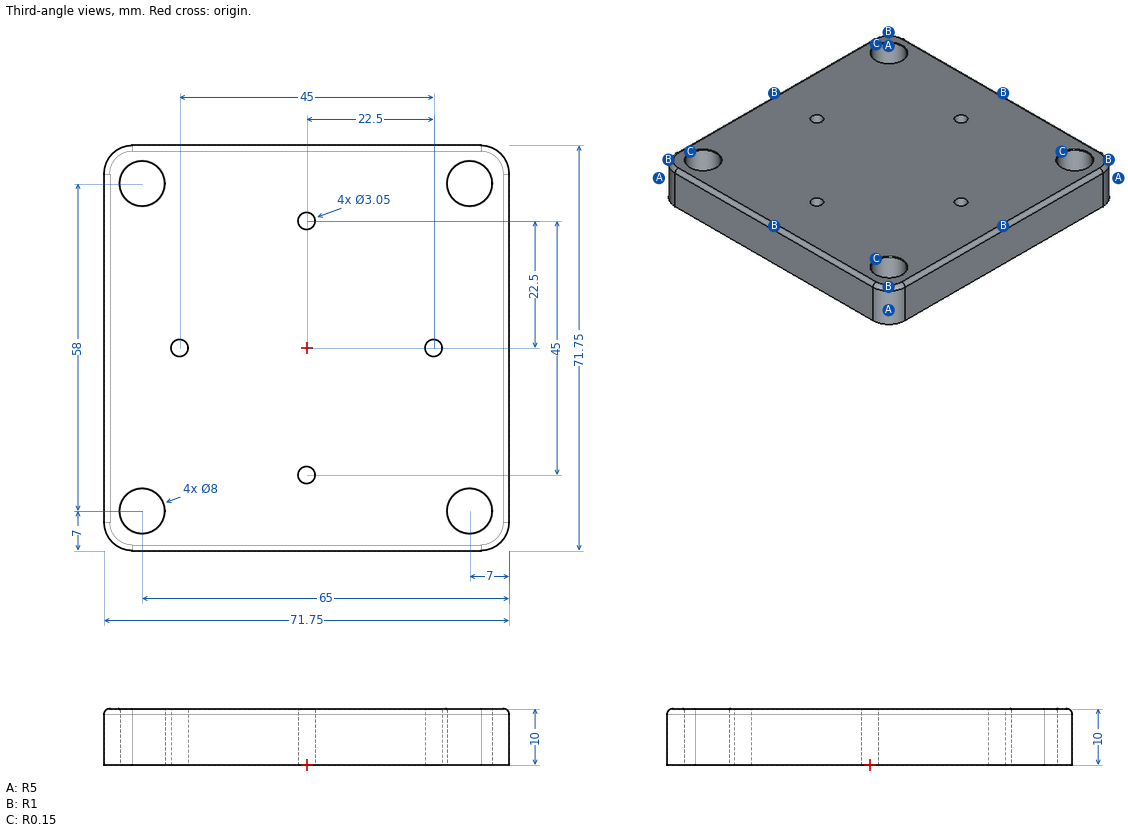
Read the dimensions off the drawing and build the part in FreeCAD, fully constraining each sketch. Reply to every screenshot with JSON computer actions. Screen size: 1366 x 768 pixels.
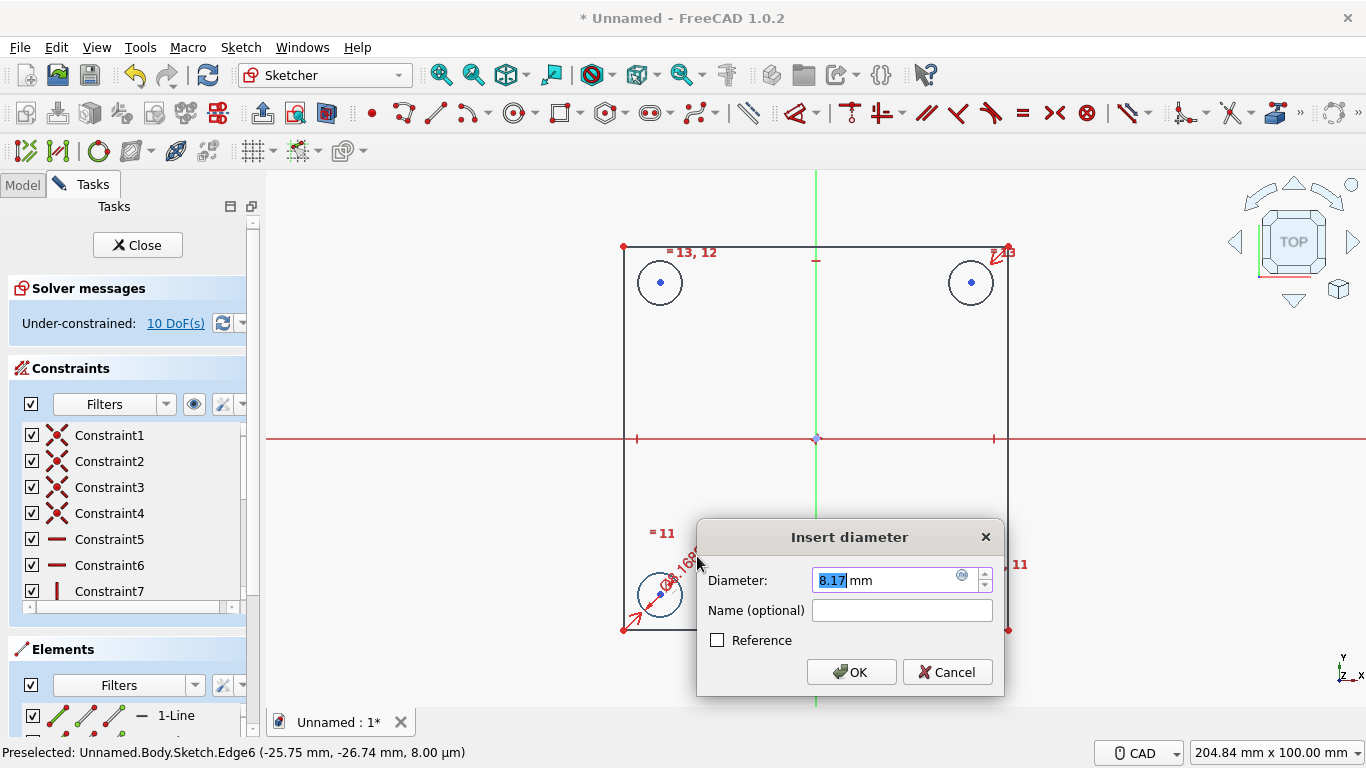
{"action": "type", "text": "8"}
{"action": "key", "text": "Return"}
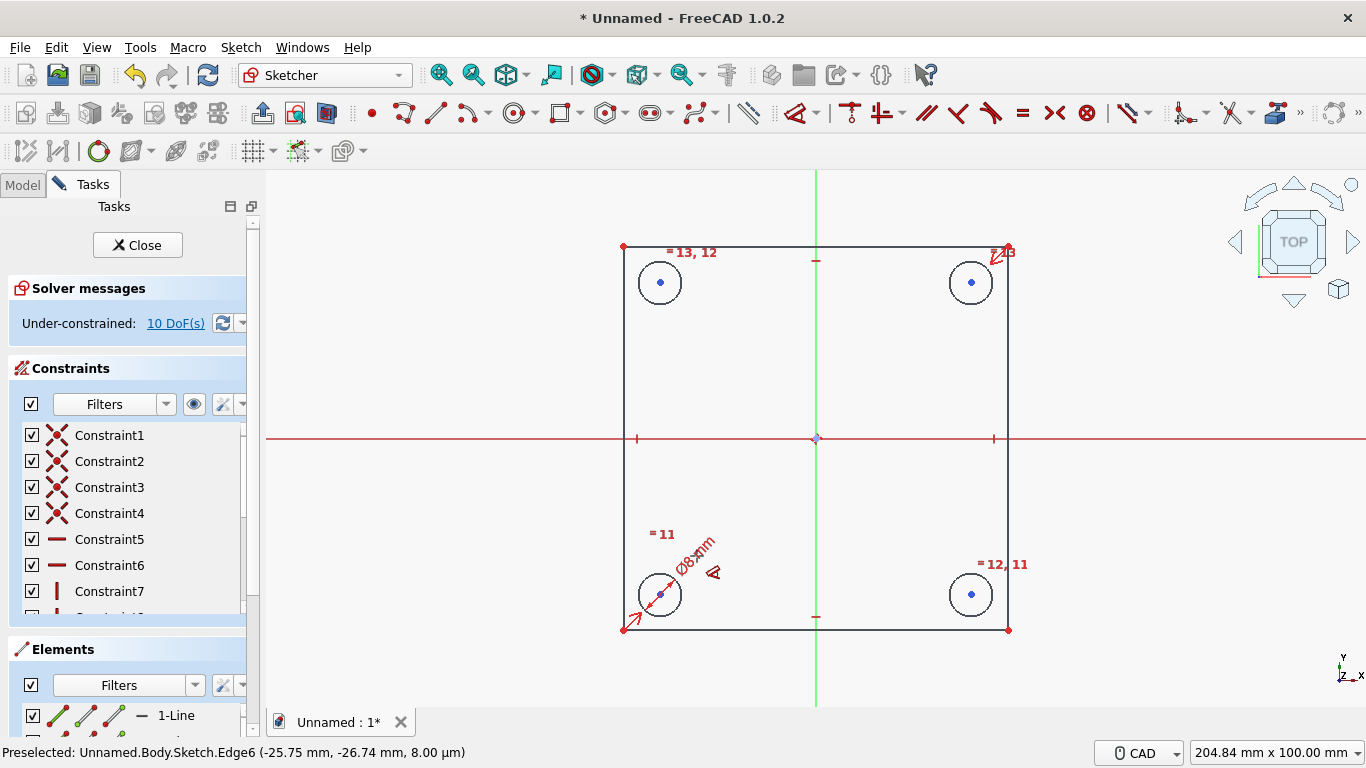
{"action": "left_click", "coordinate": [624, 630]}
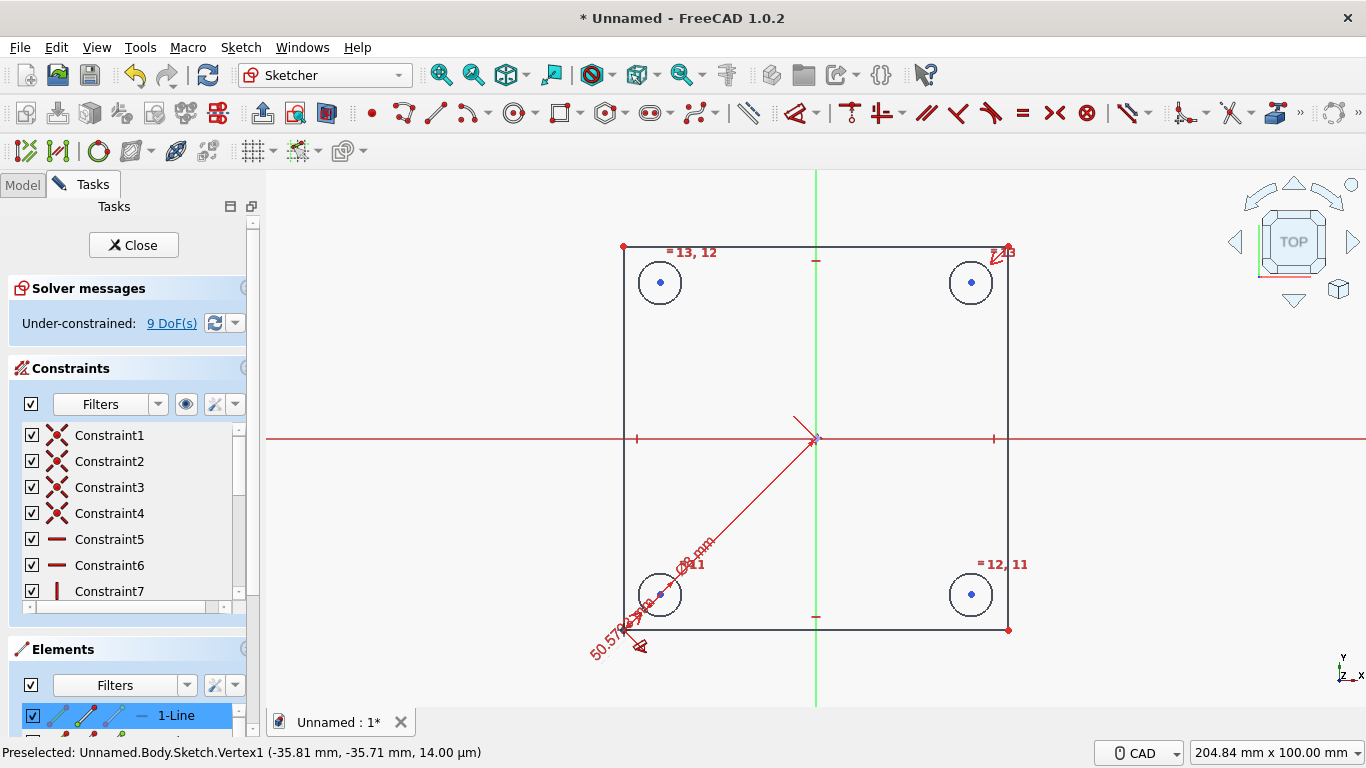
{"action": "left_click", "coordinate": [660, 595]}
{"action": "left_click", "coordinate": [590, 613]}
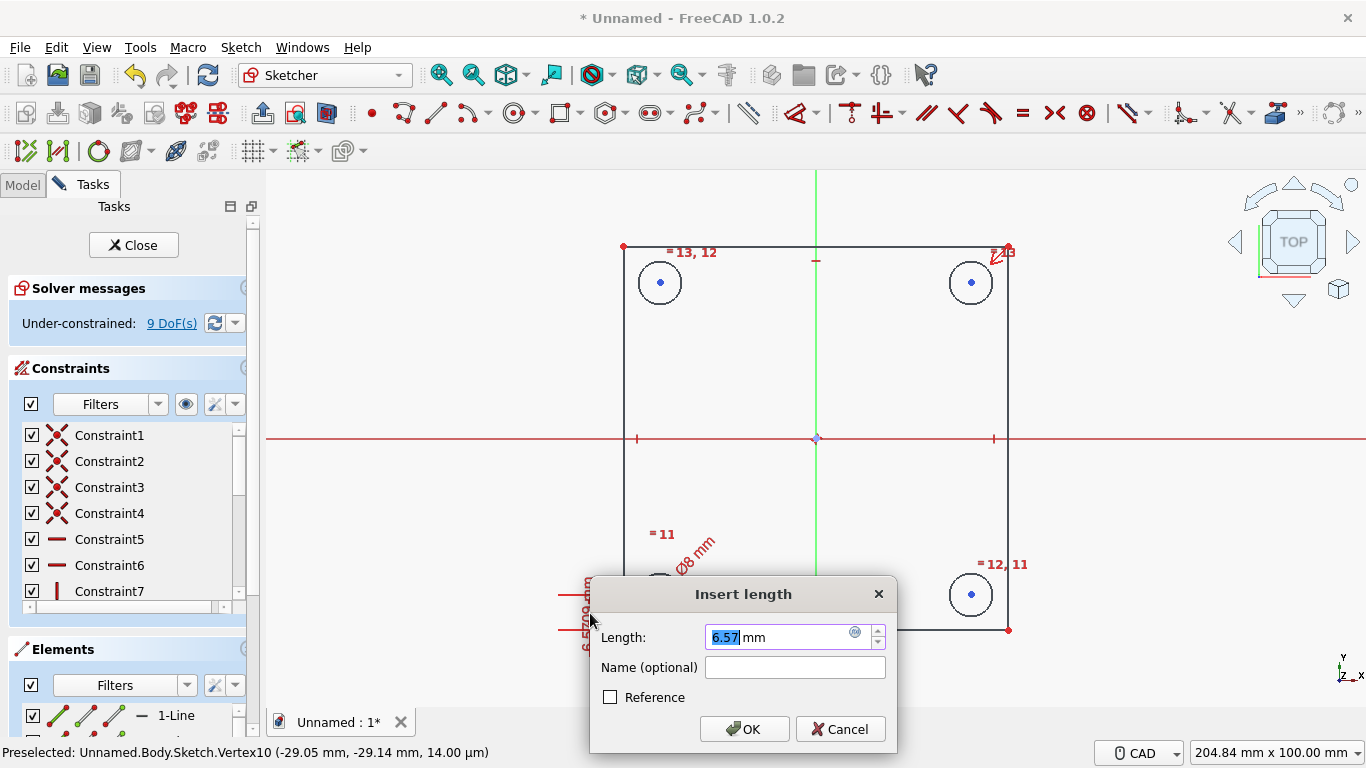
{"action": "type", "text": "7"}
{"action": "key", "text": "Return"}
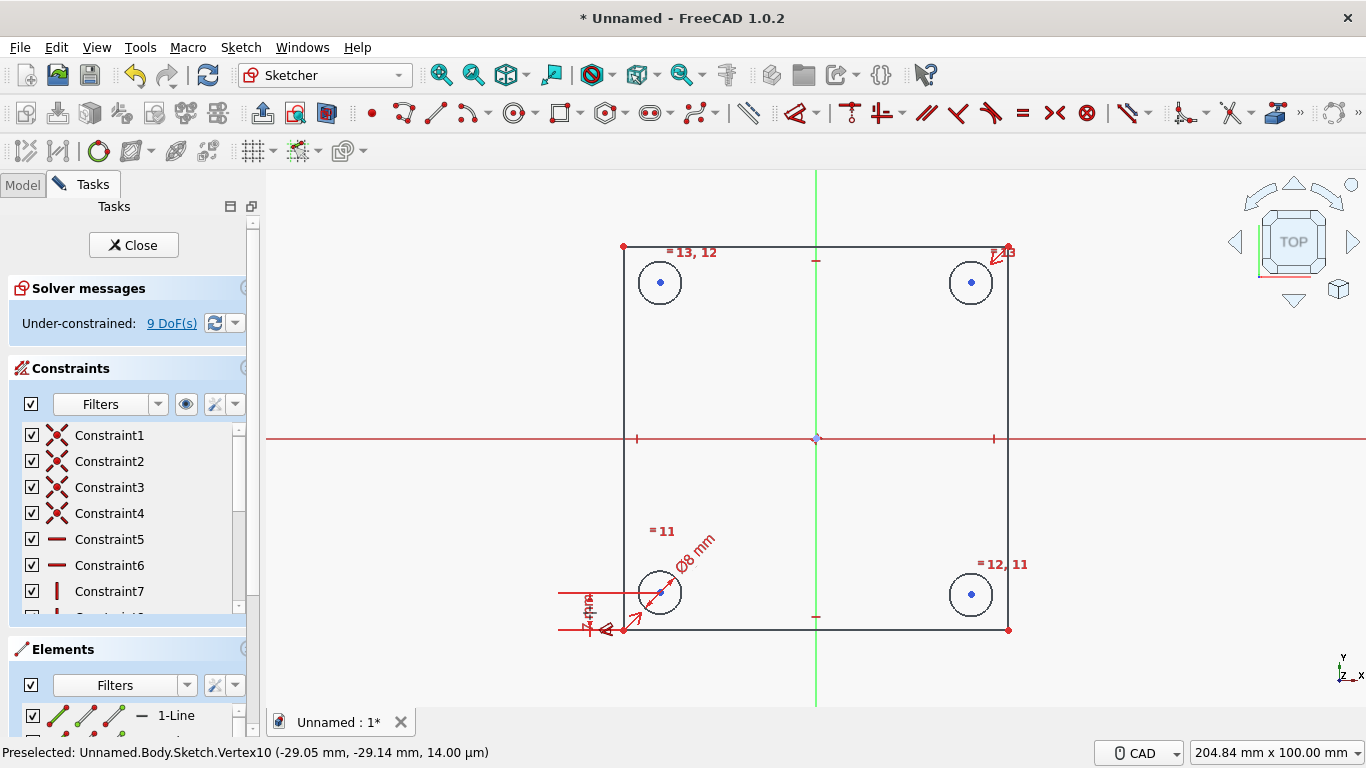
{"action": "left_click", "coordinate": [1008, 630]}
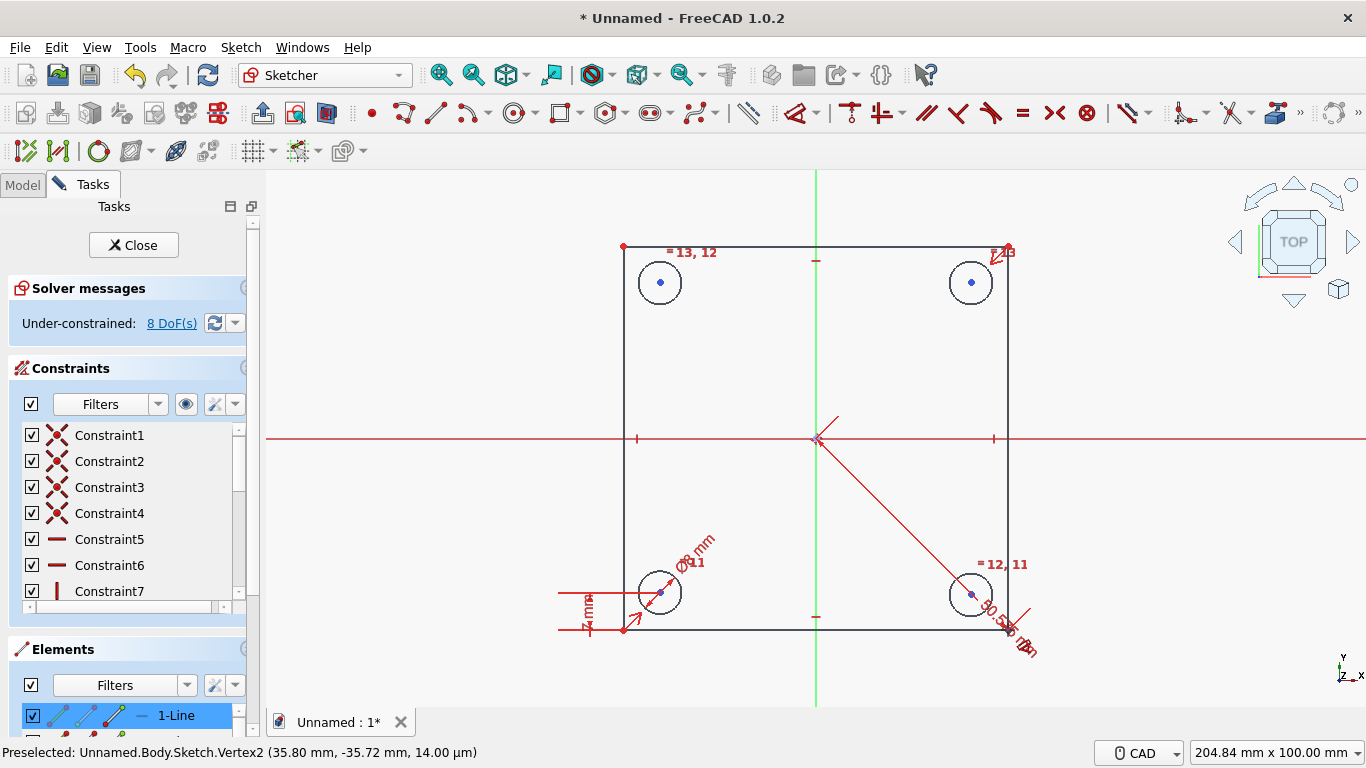
{"action": "left_click", "coordinate": [971, 595]}
{"action": "left_click", "coordinate": [990, 664]}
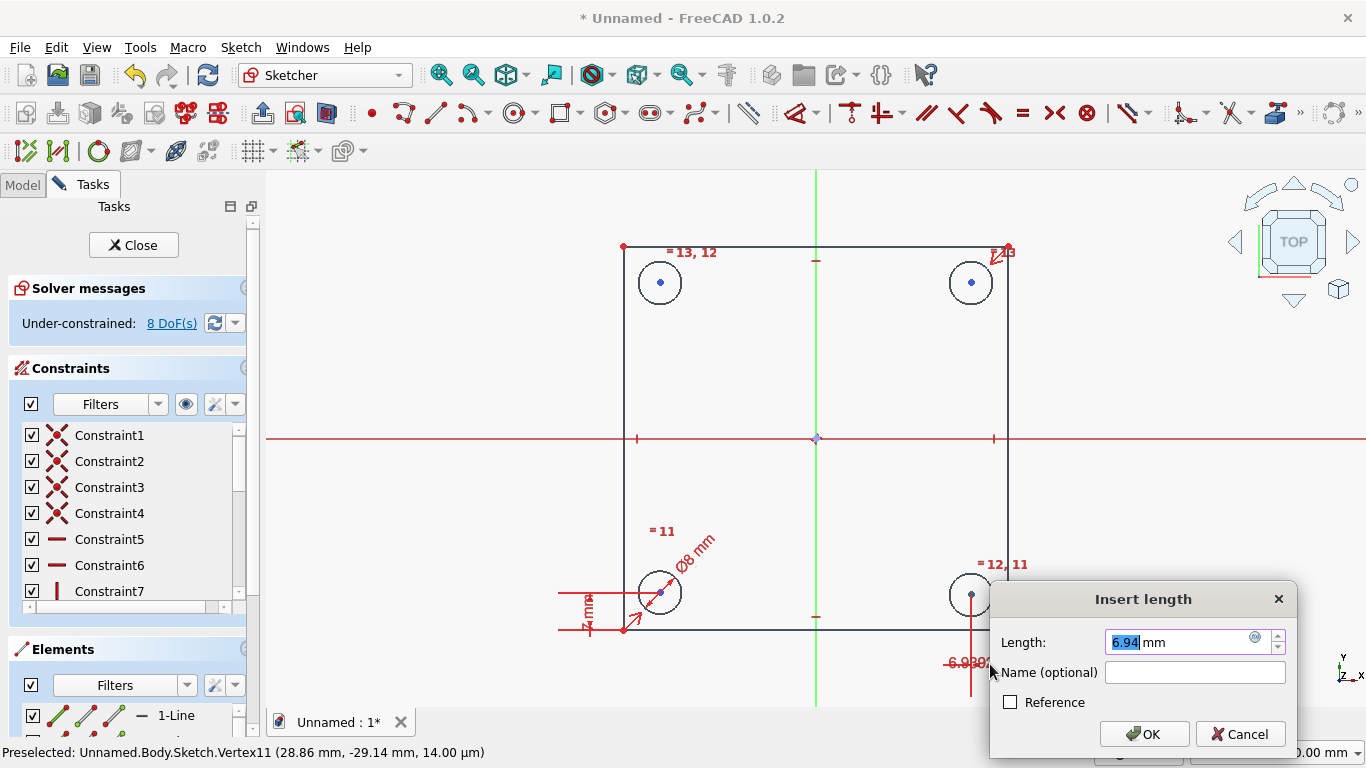
{"action": "type", "text": "7"}
{"action": "key", "text": "Return"}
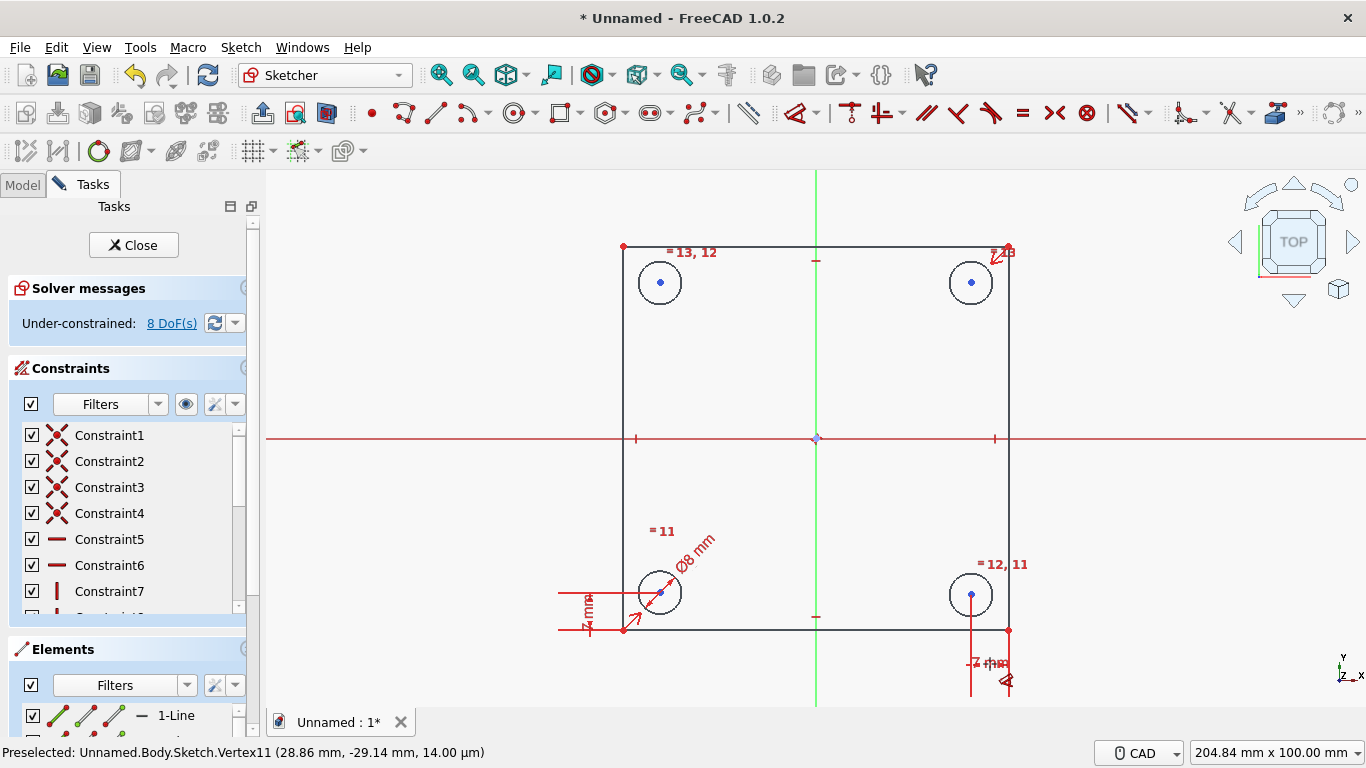
{"action": "left_click", "coordinate": [1009, 630]}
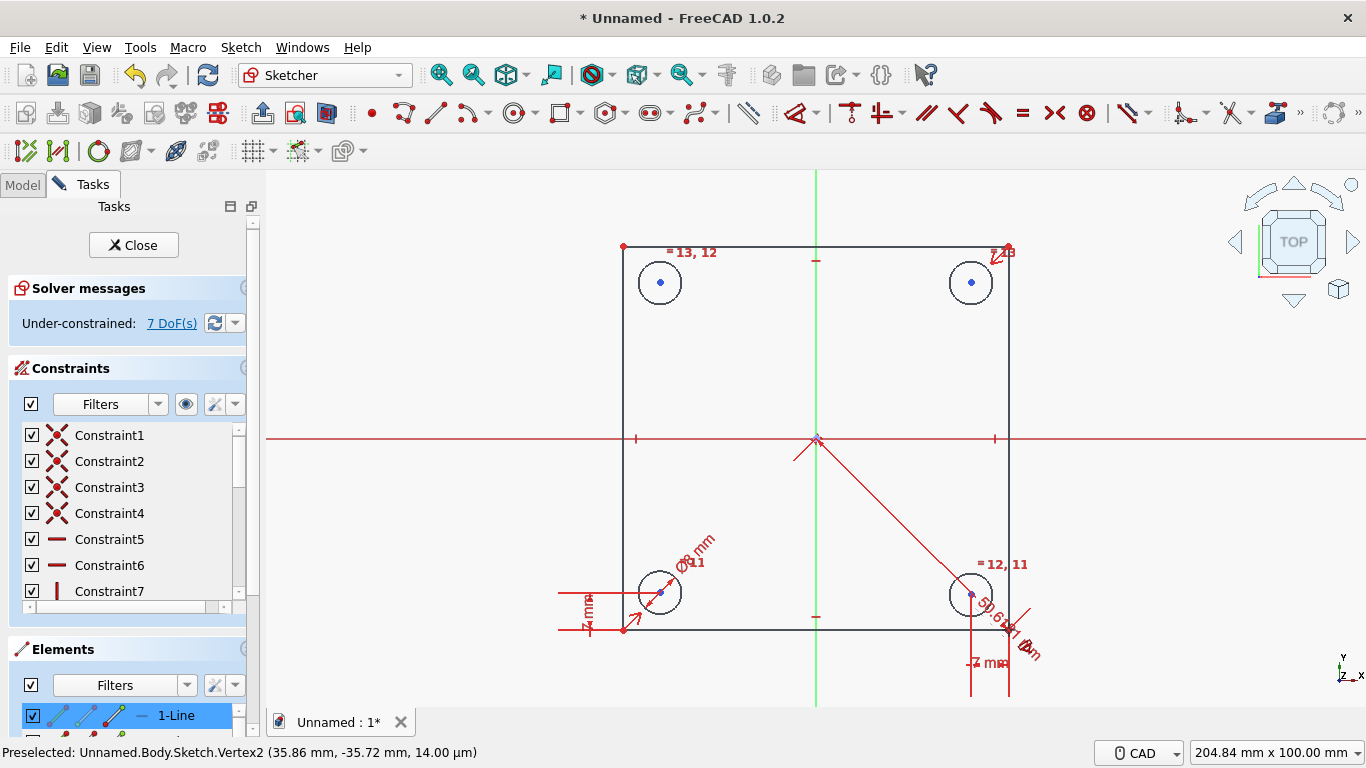
{"action": "left_click", "coordinate": [971, 595]}
{"action": "left_click", "coordinate": [1043, 613]}